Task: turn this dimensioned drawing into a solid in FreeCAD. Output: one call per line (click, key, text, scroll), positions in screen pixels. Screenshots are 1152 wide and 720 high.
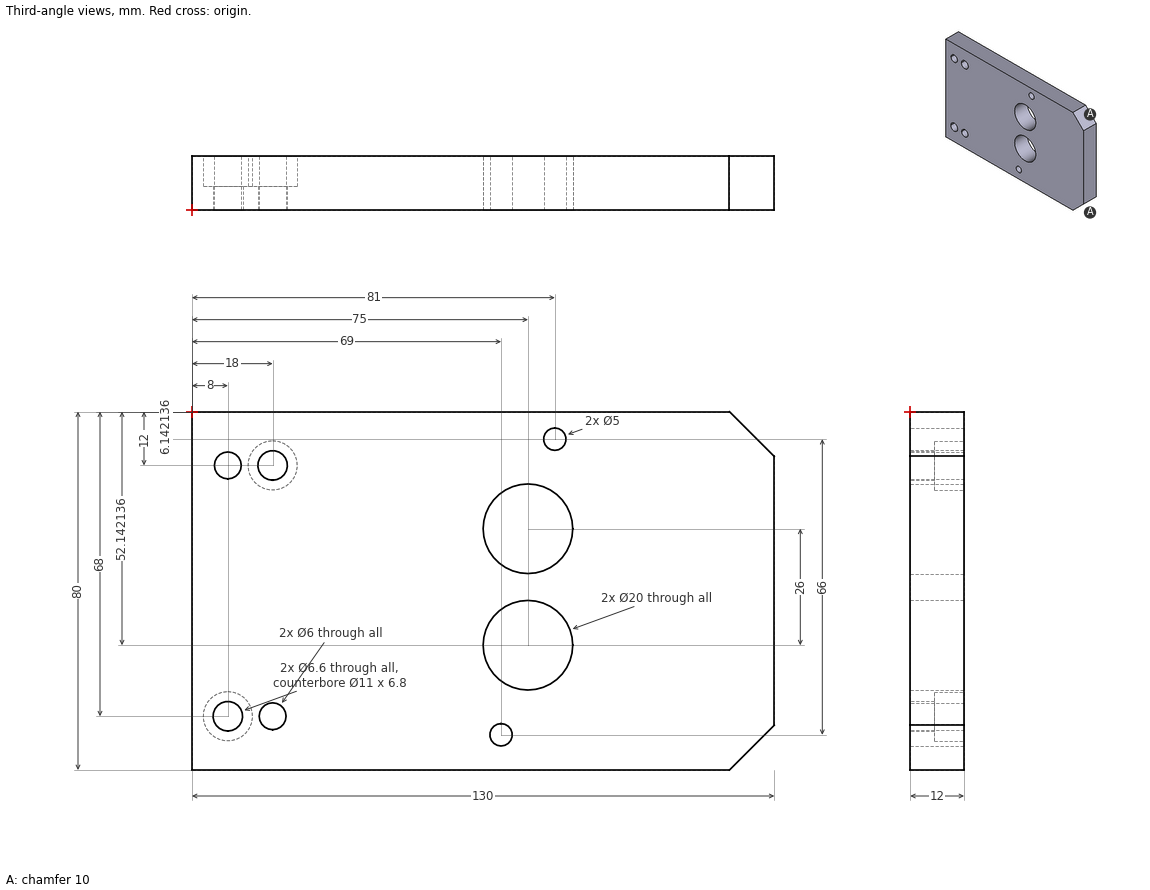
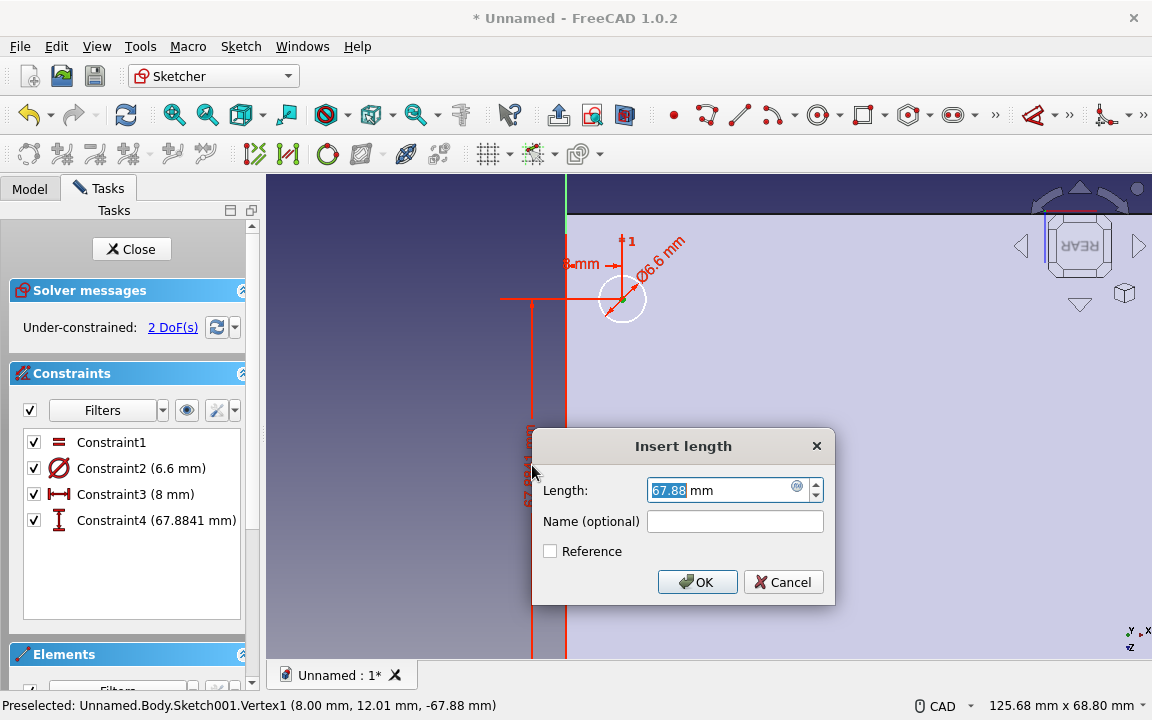
text(68)
key(Return)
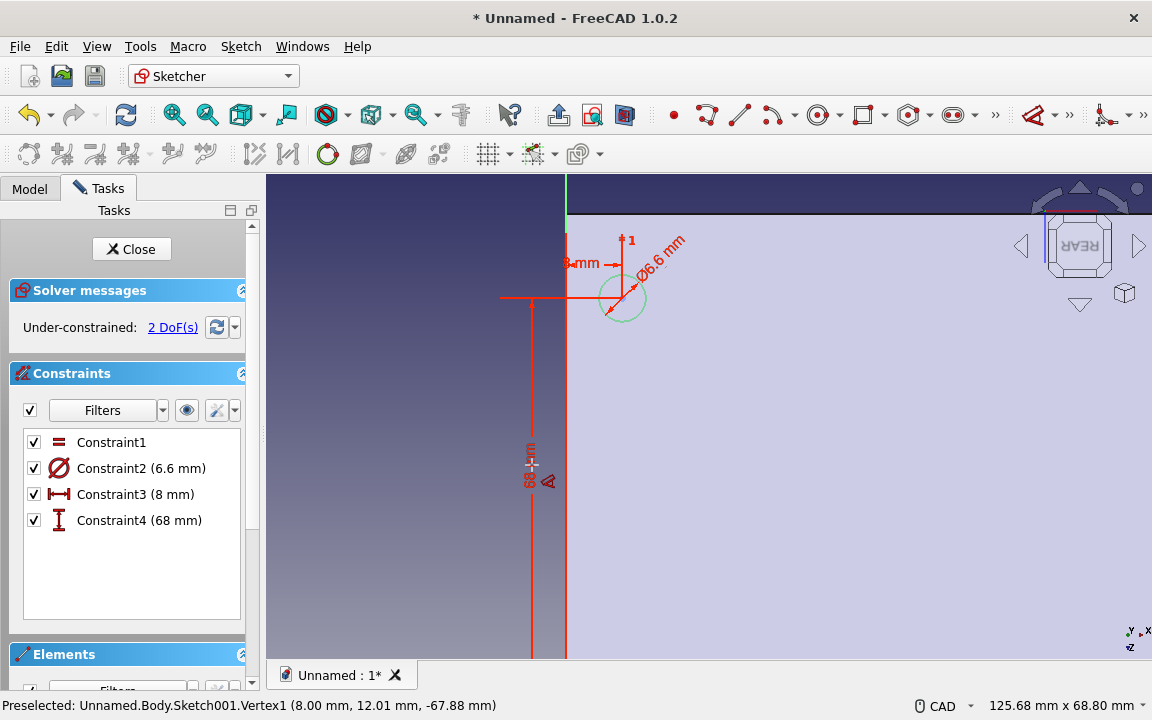
scroll(640, 283, down, 3)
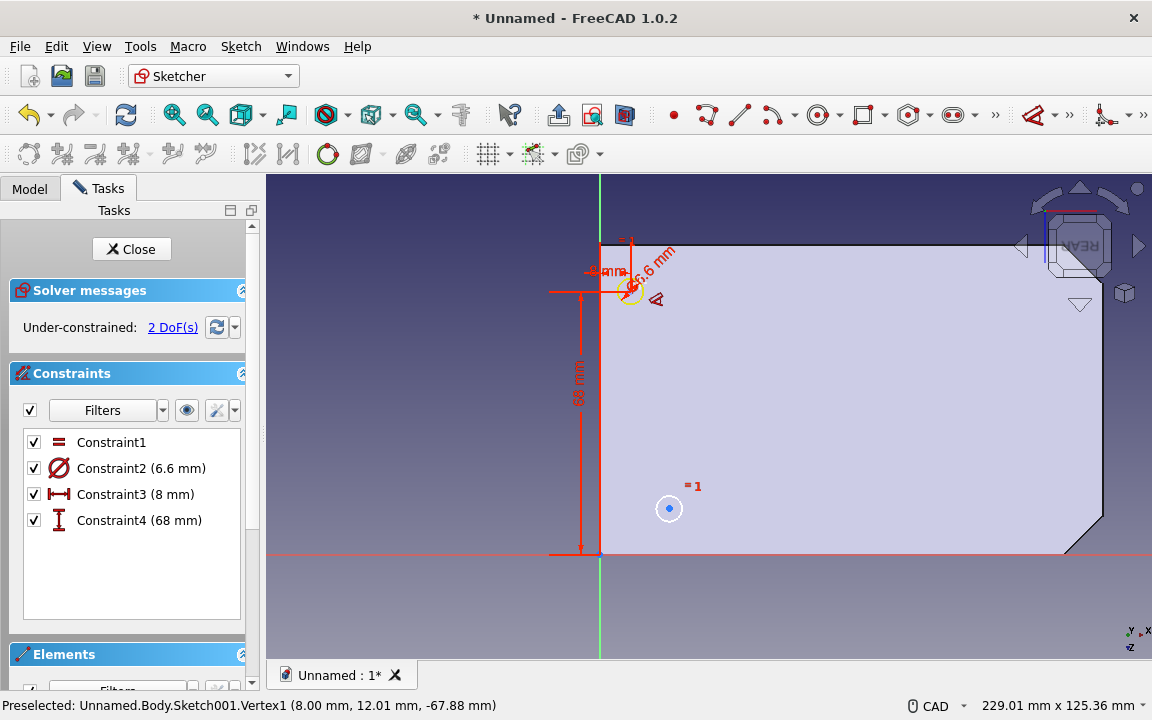
click(669, 509)
click(634, 589)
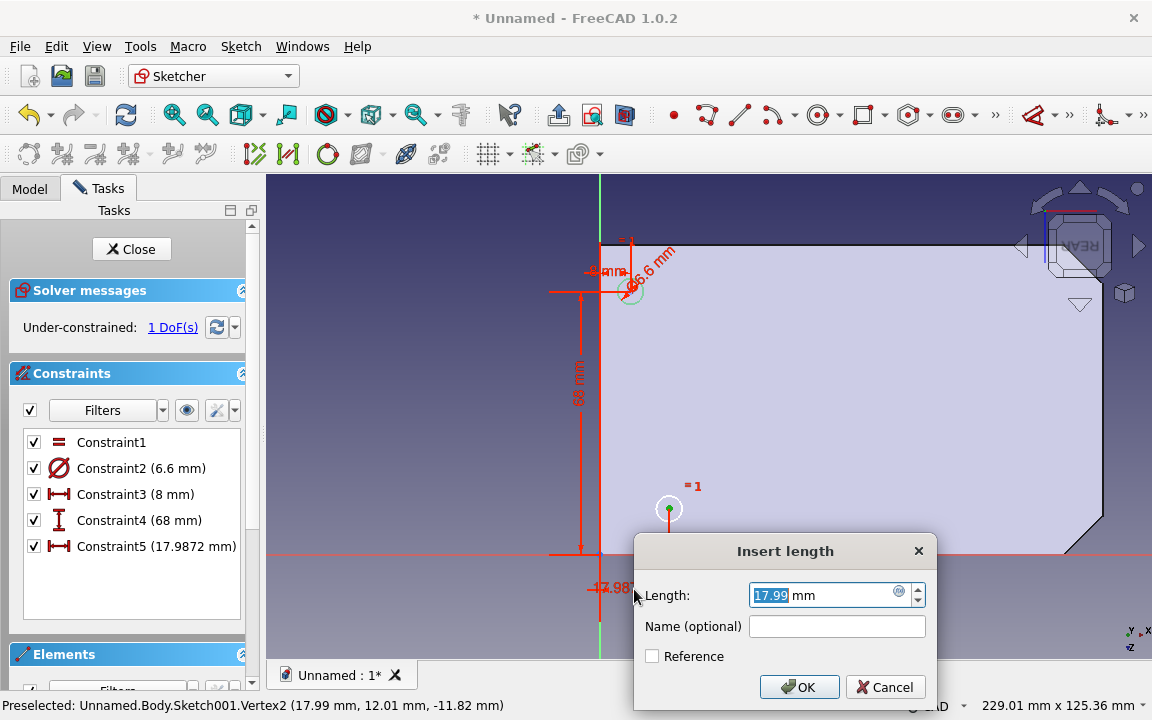
text(18)
key(Return)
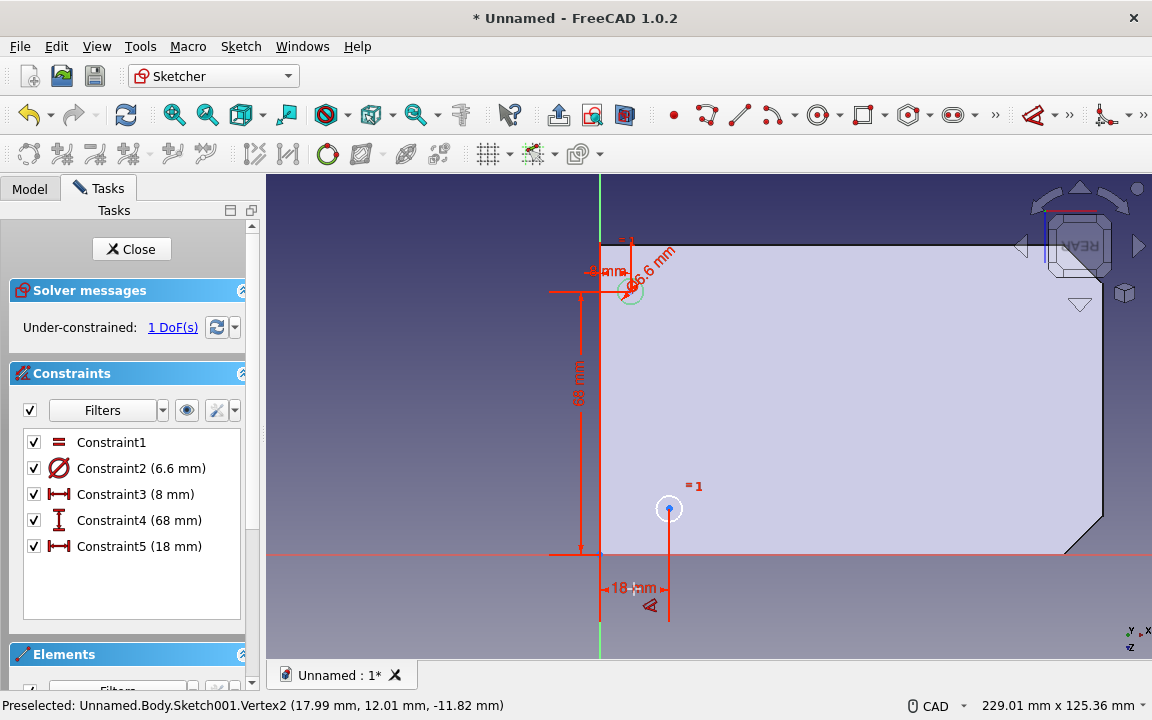
click(669, 509)
click(566, 532)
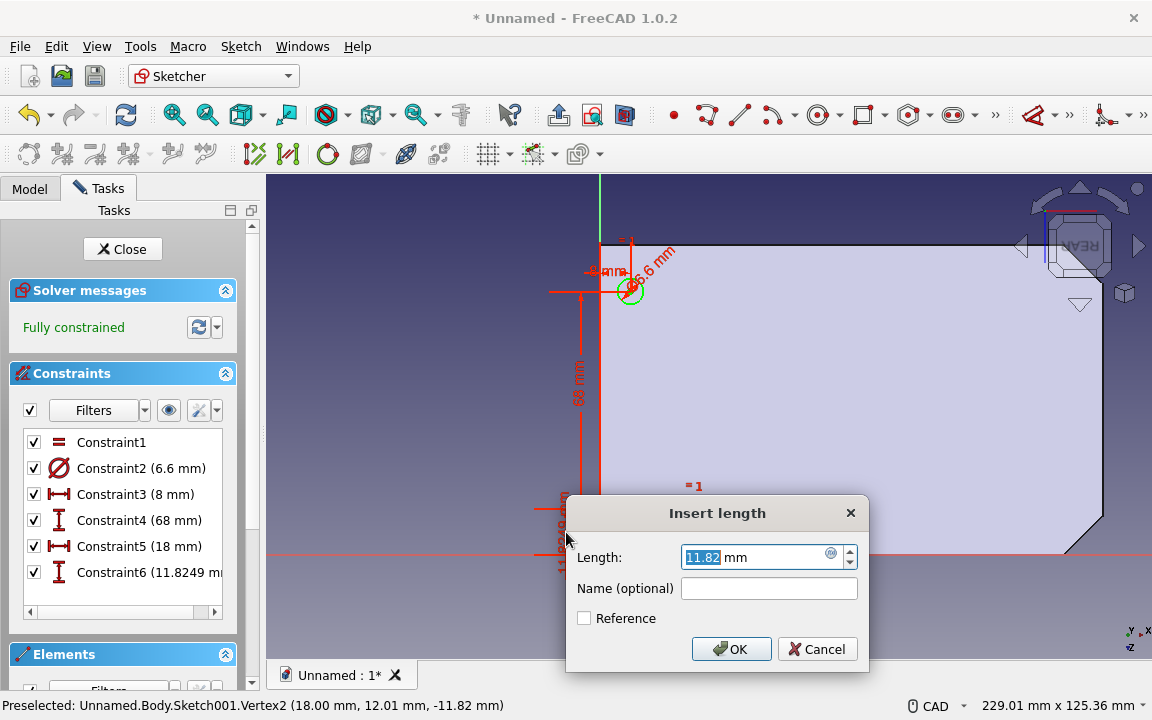
text(12)
key(Return)
key(Escape)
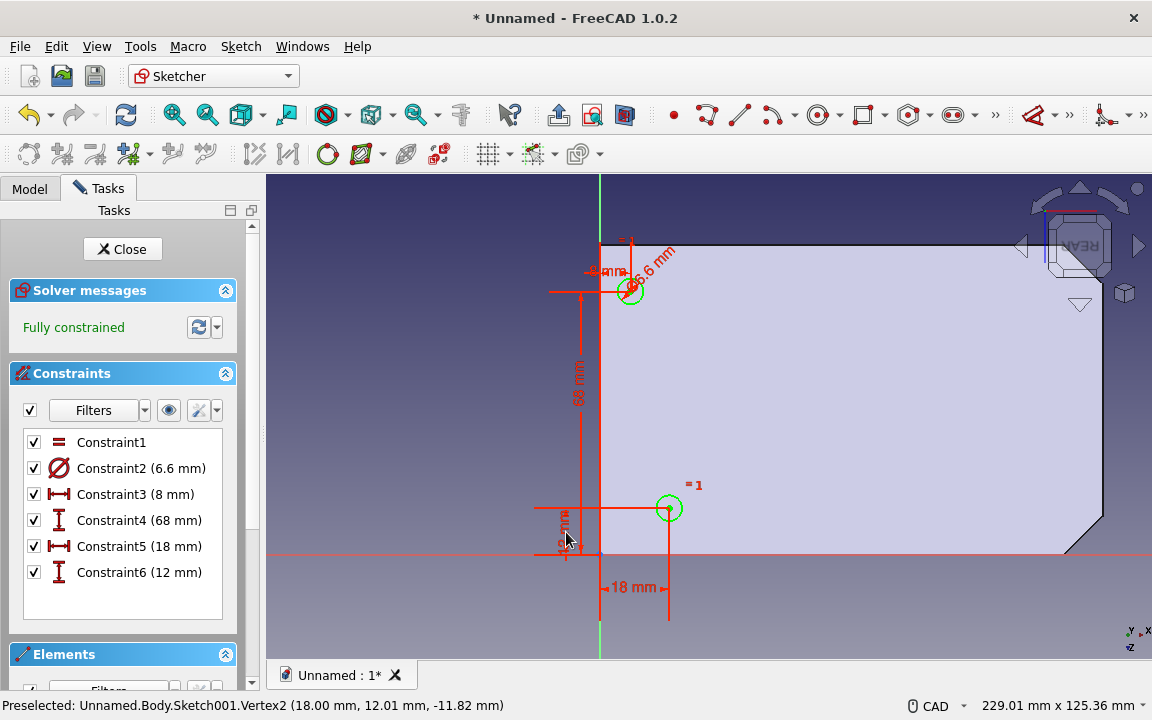
click(123, 249)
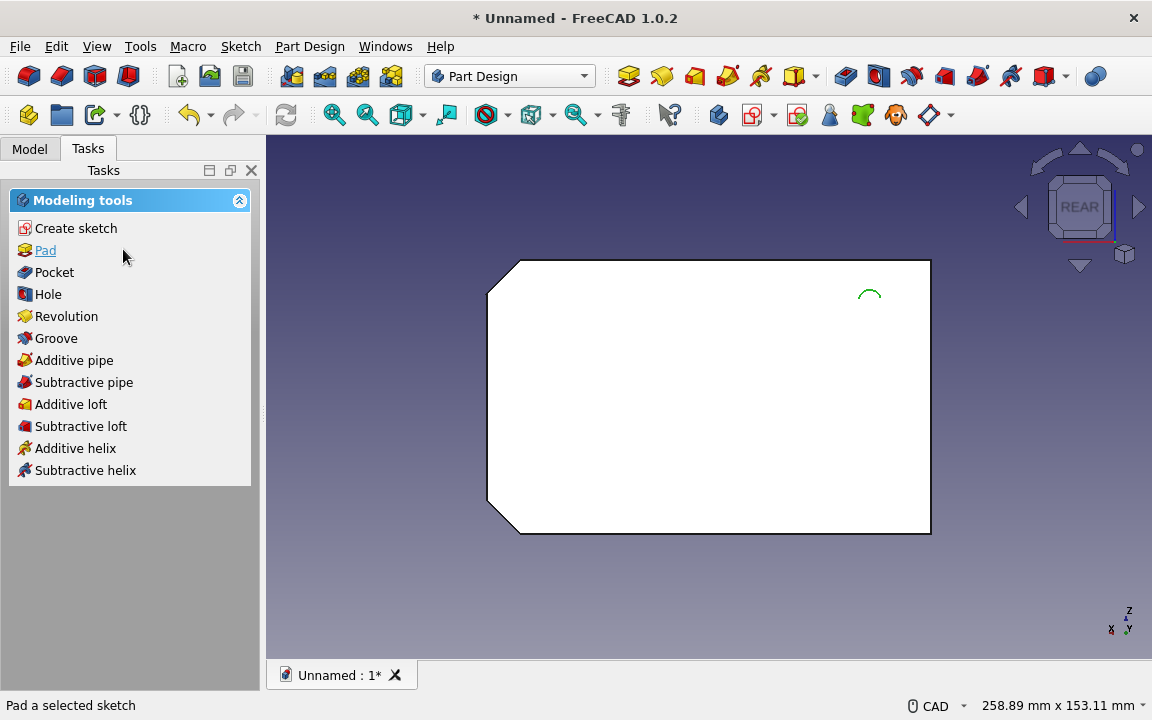
click(879, 76)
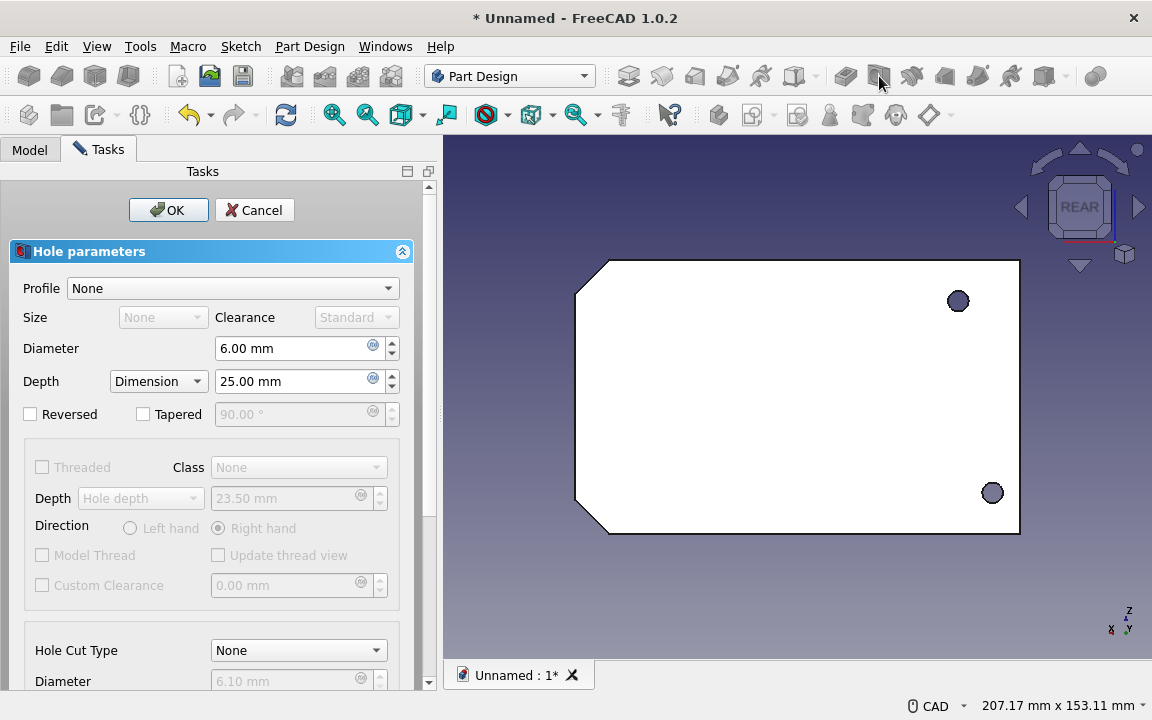
triple_click(300, 348)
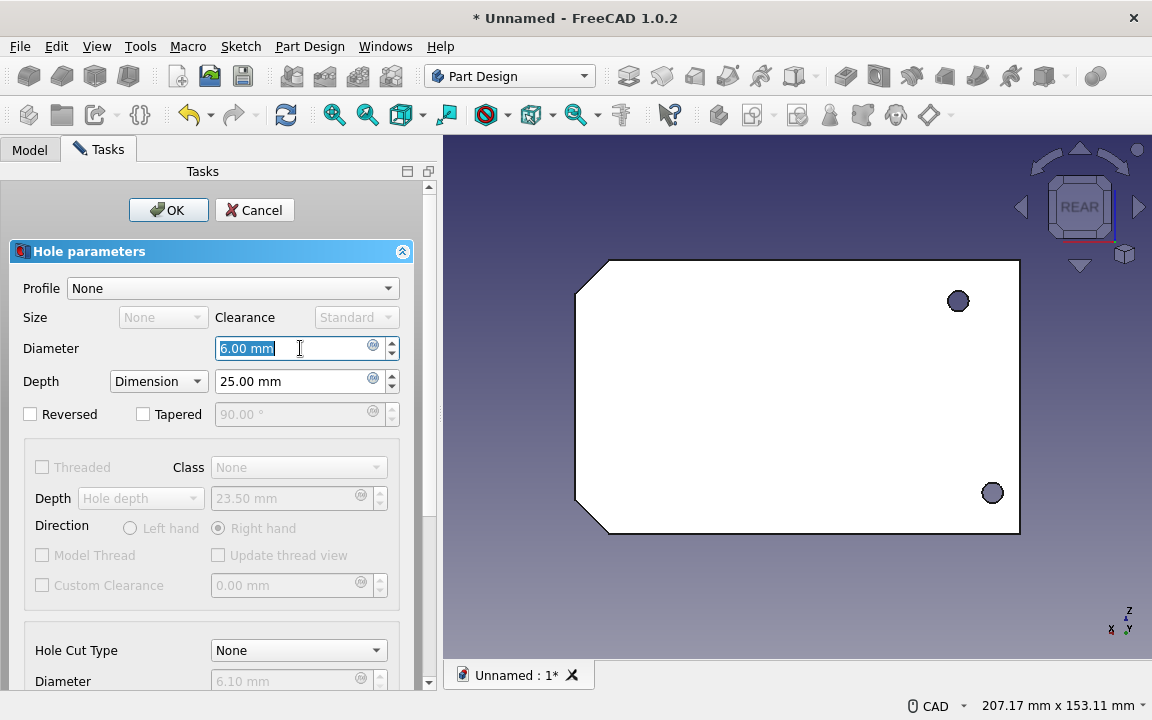
text(6.6)
key(Tab)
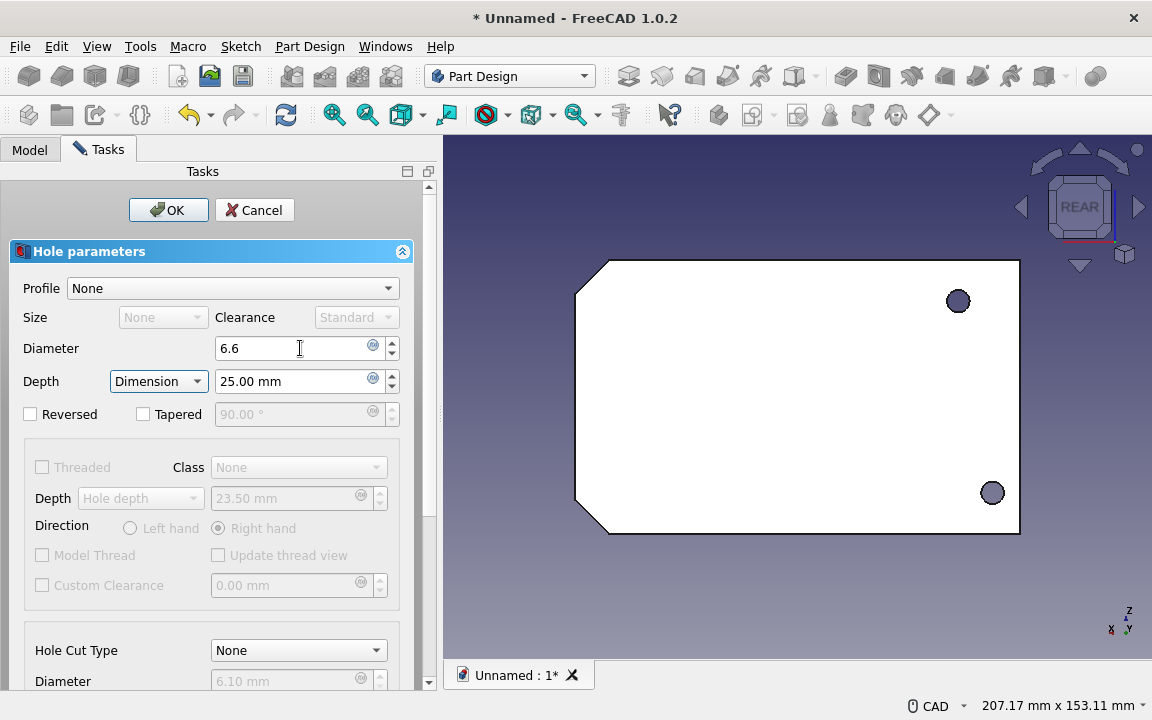
click(160, 382)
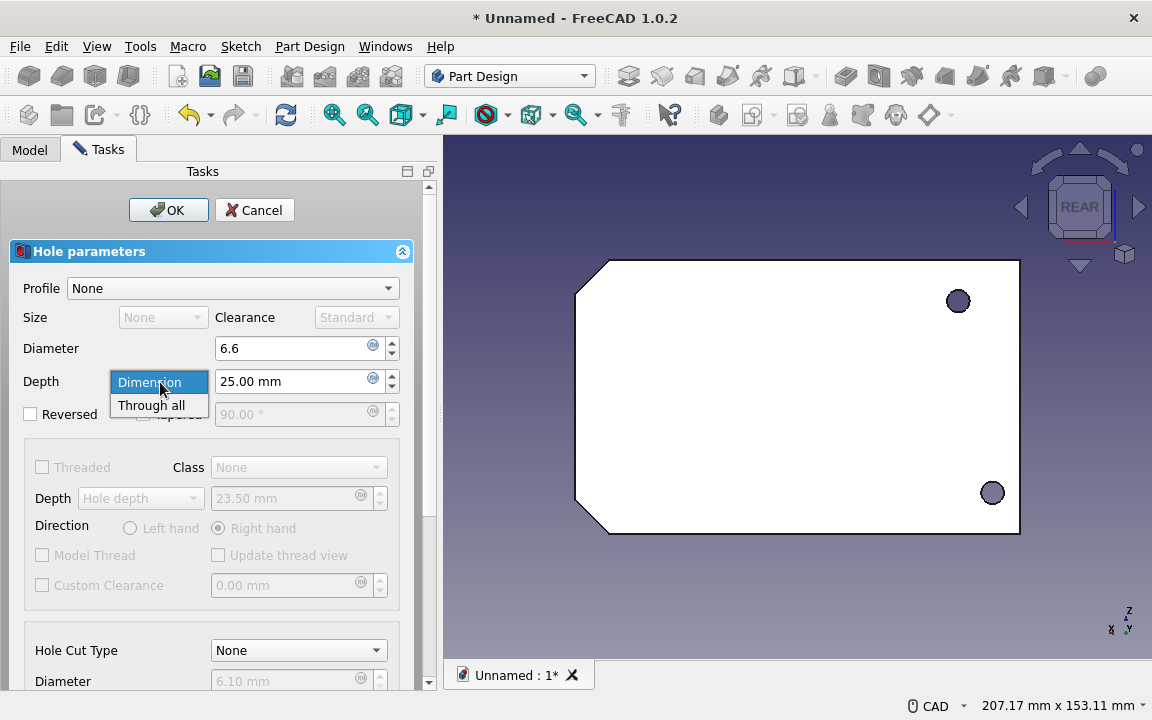
click(158, 406)